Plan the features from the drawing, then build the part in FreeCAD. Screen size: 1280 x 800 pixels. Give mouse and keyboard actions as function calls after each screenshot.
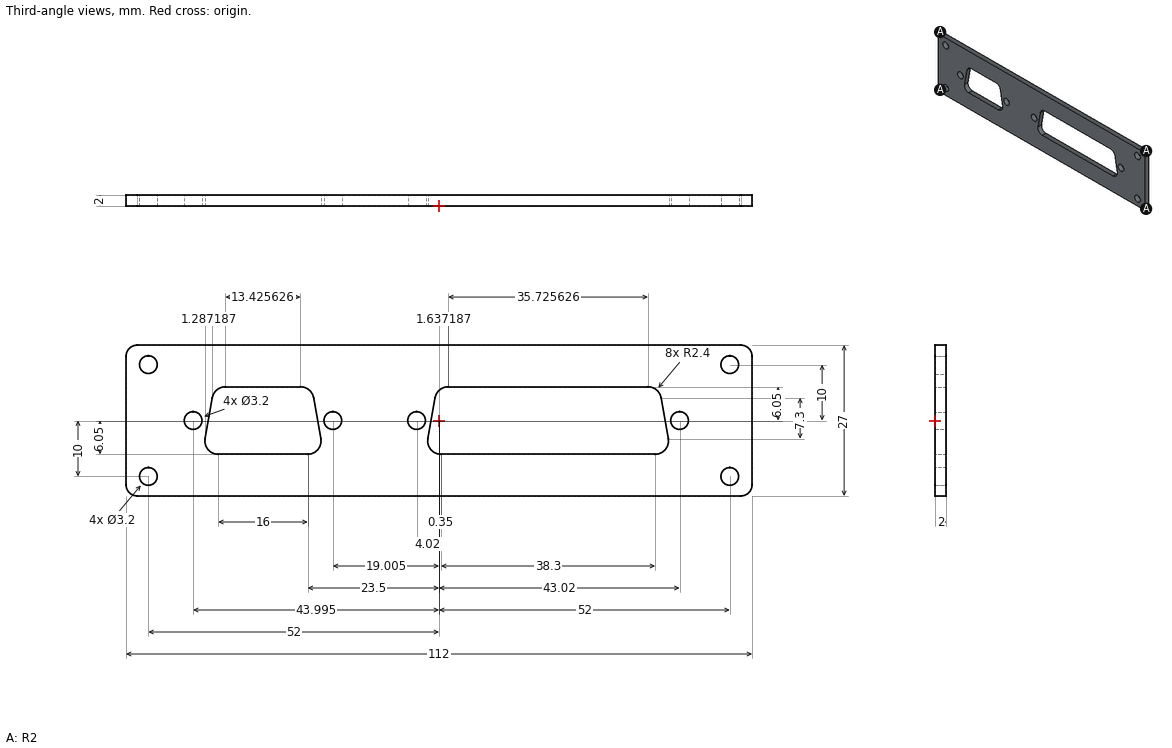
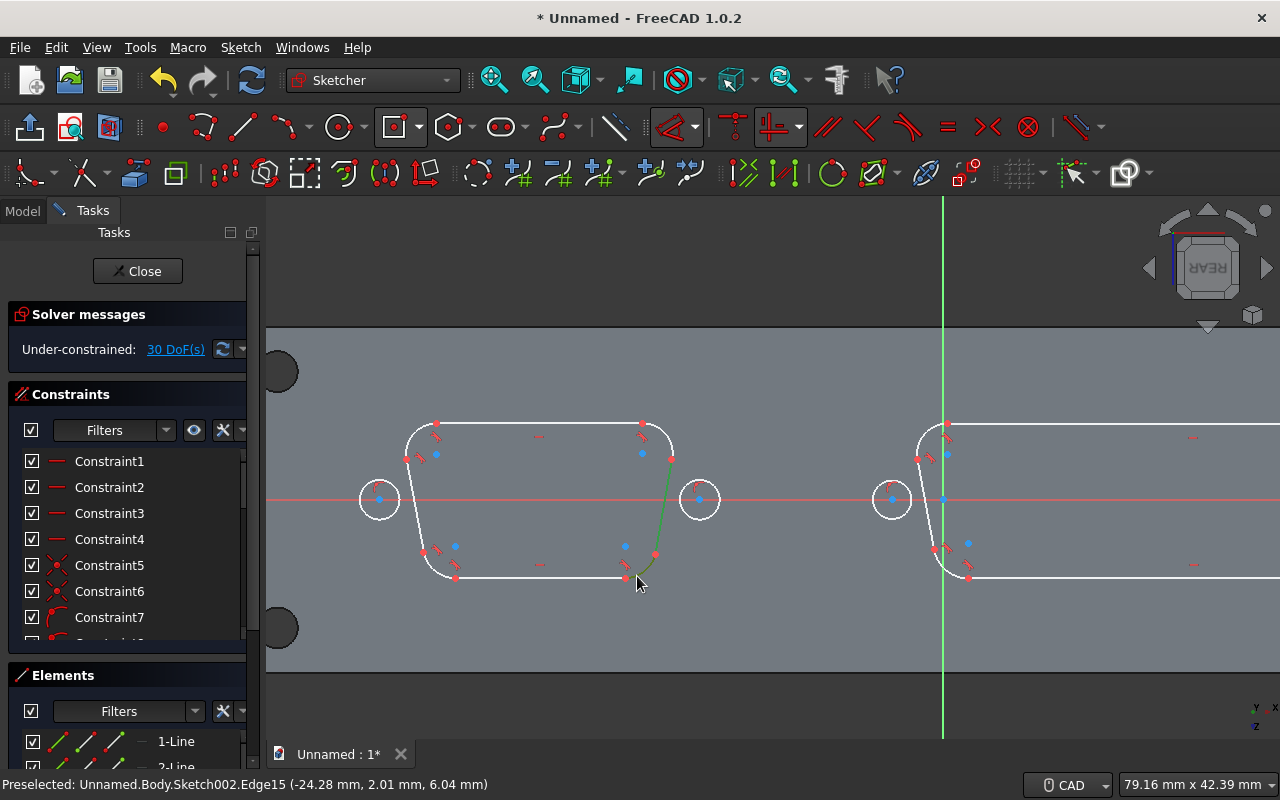
click(908, 128)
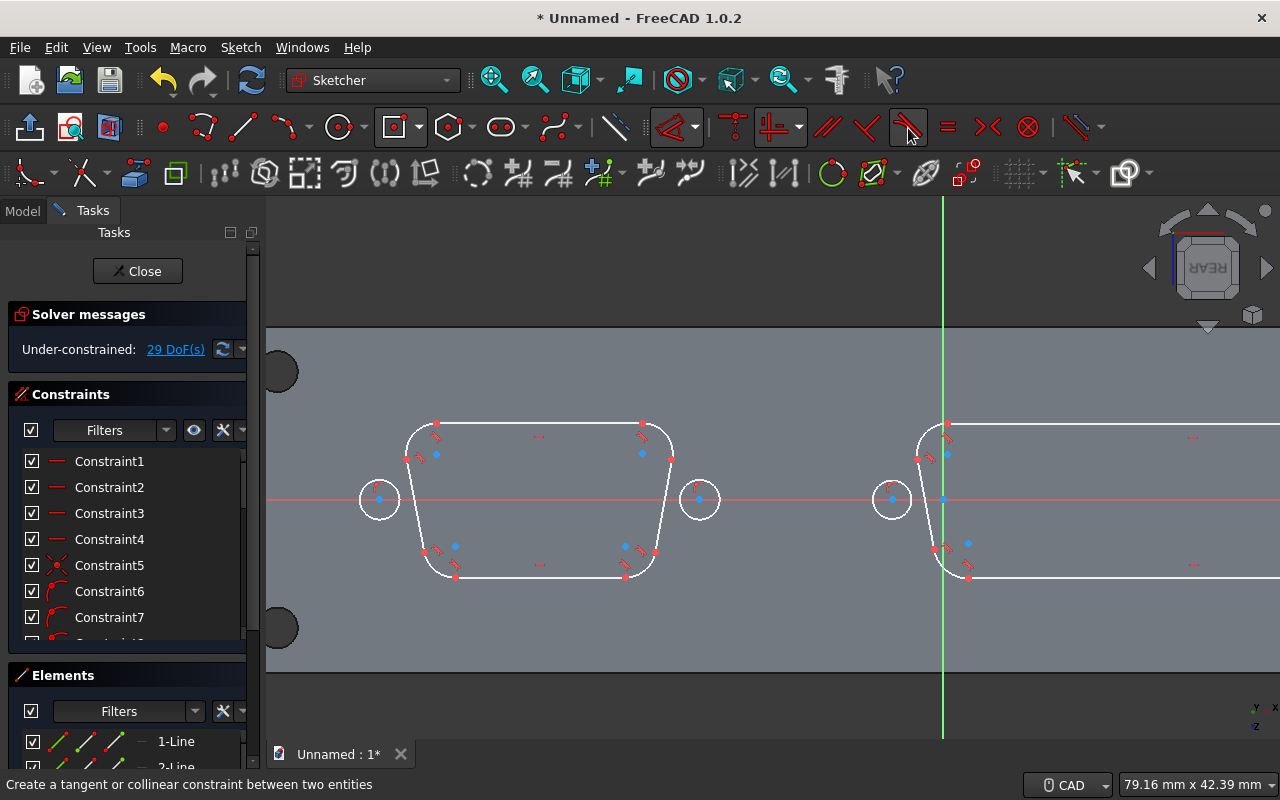
click(660, 525)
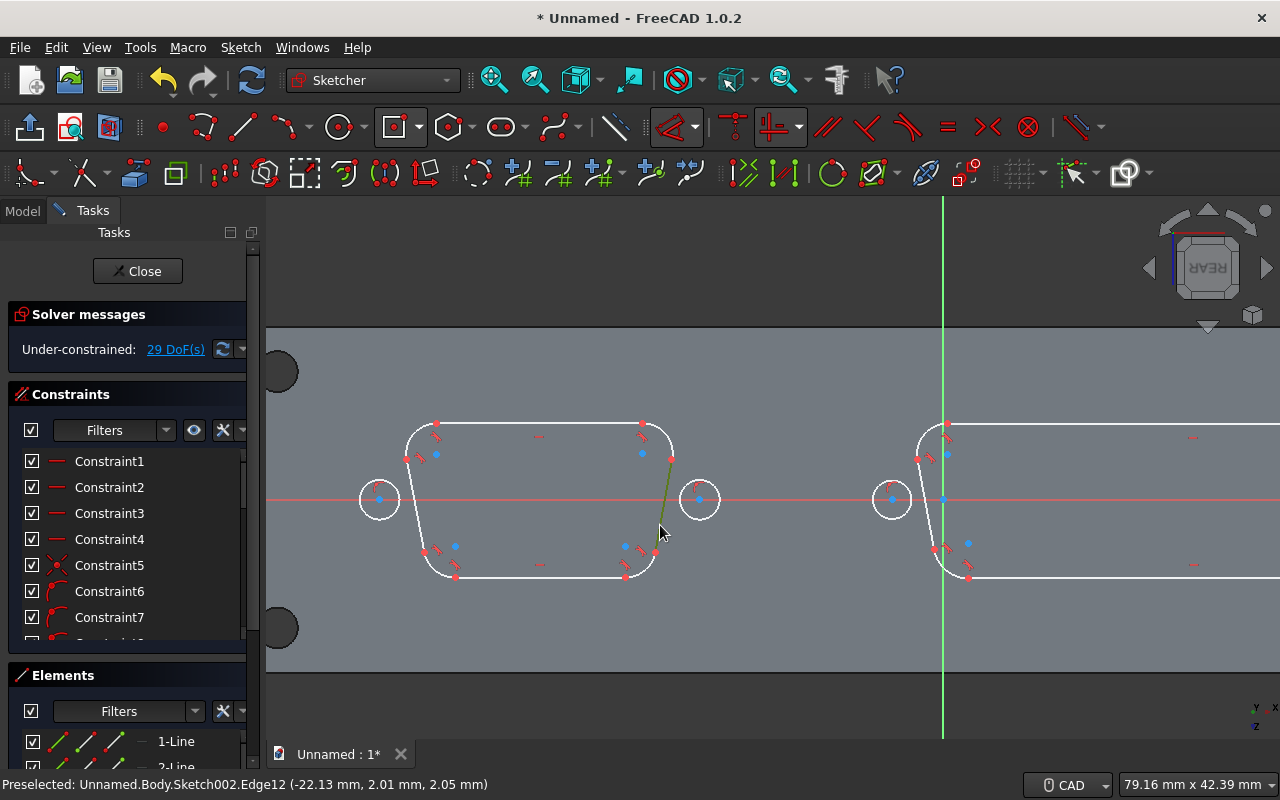
click(671, 444)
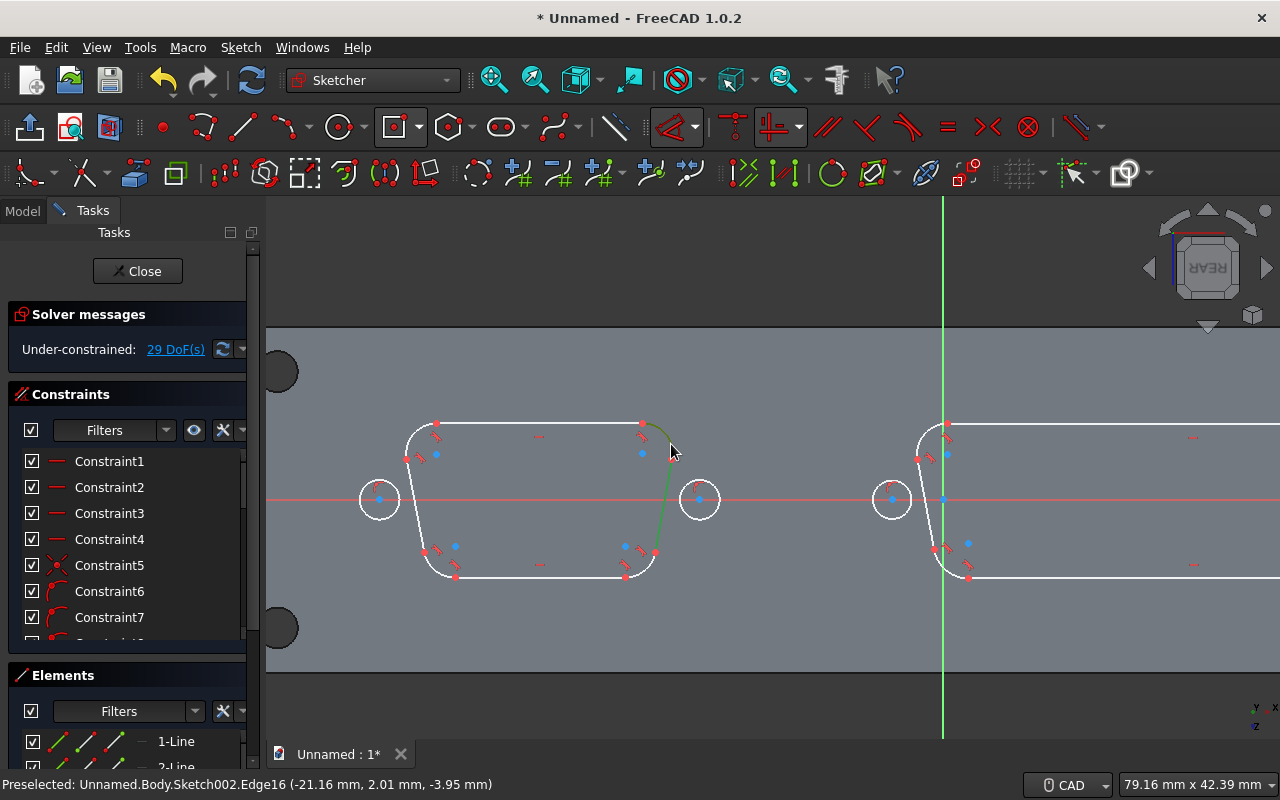
key(t)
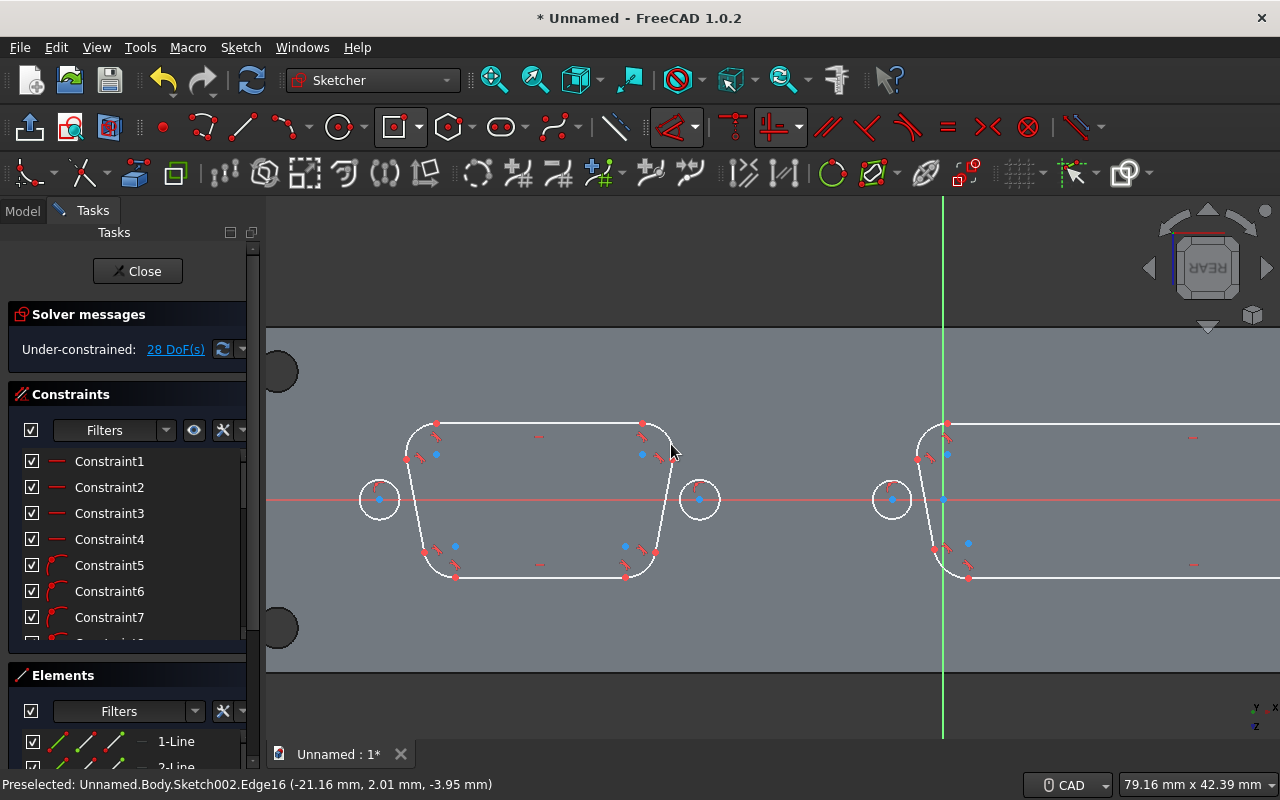
scroll(421, 428, down, 3)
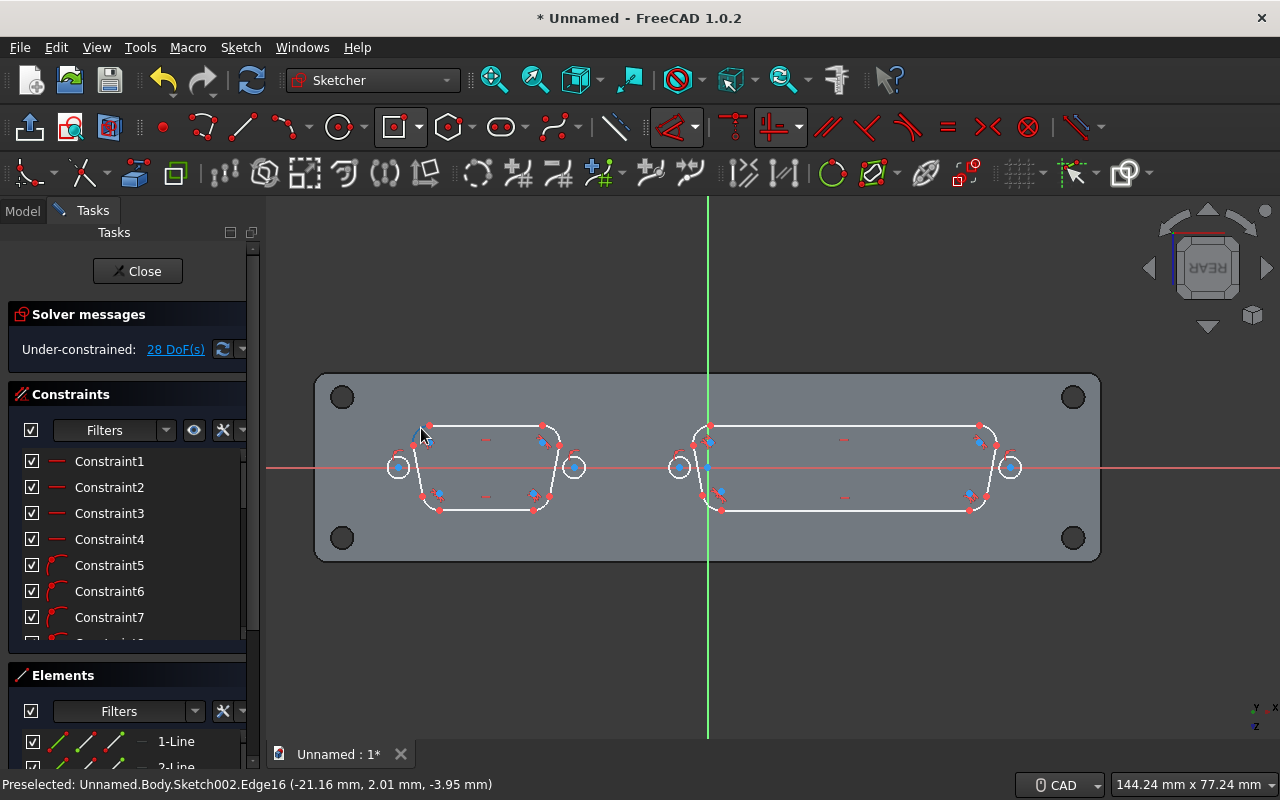
scroll(977, 509, up, 4)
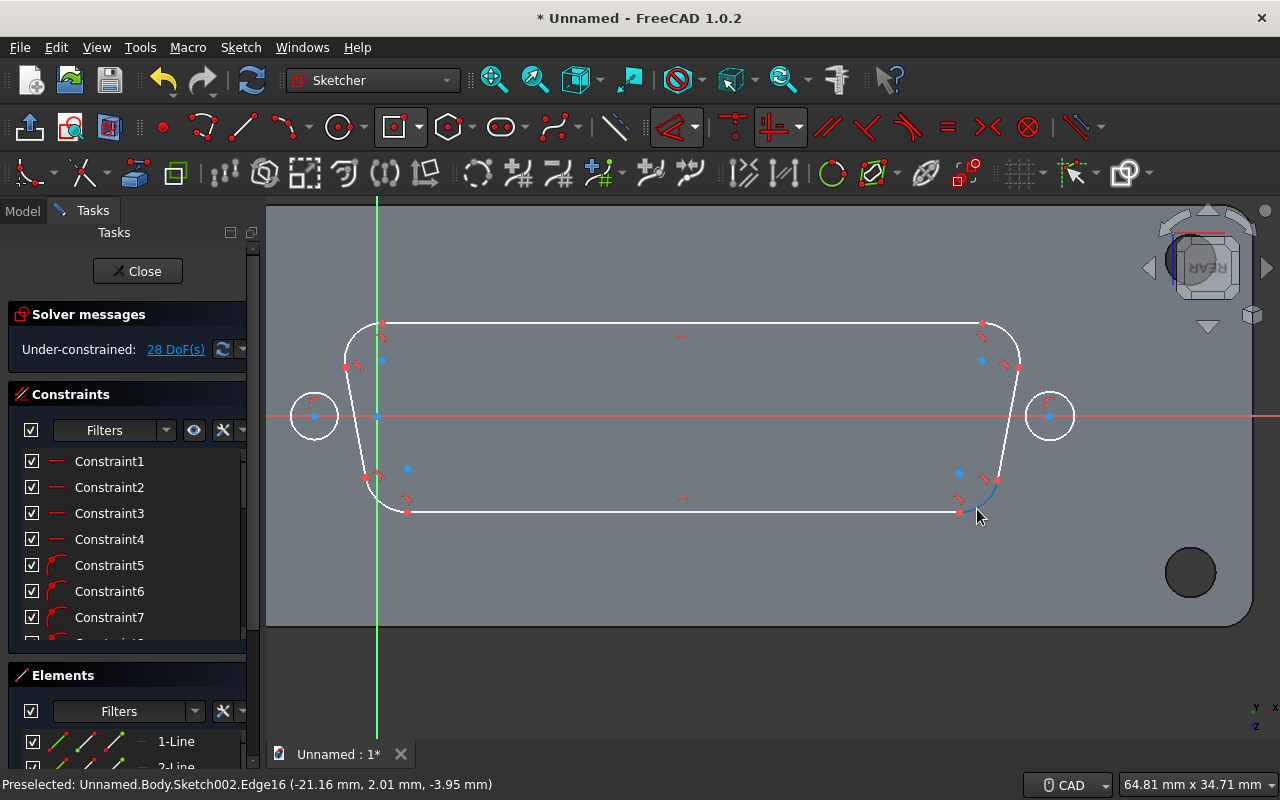
click(975, 509)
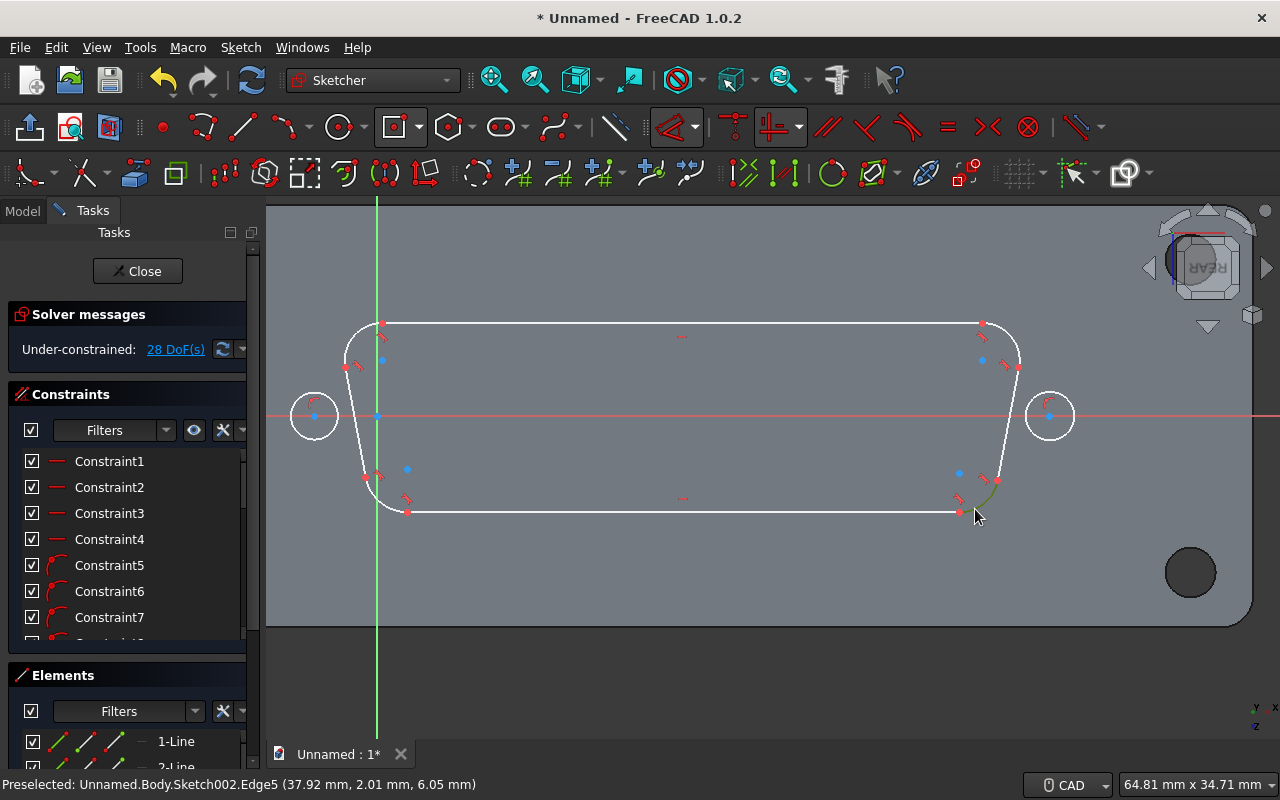
click(1017, 348)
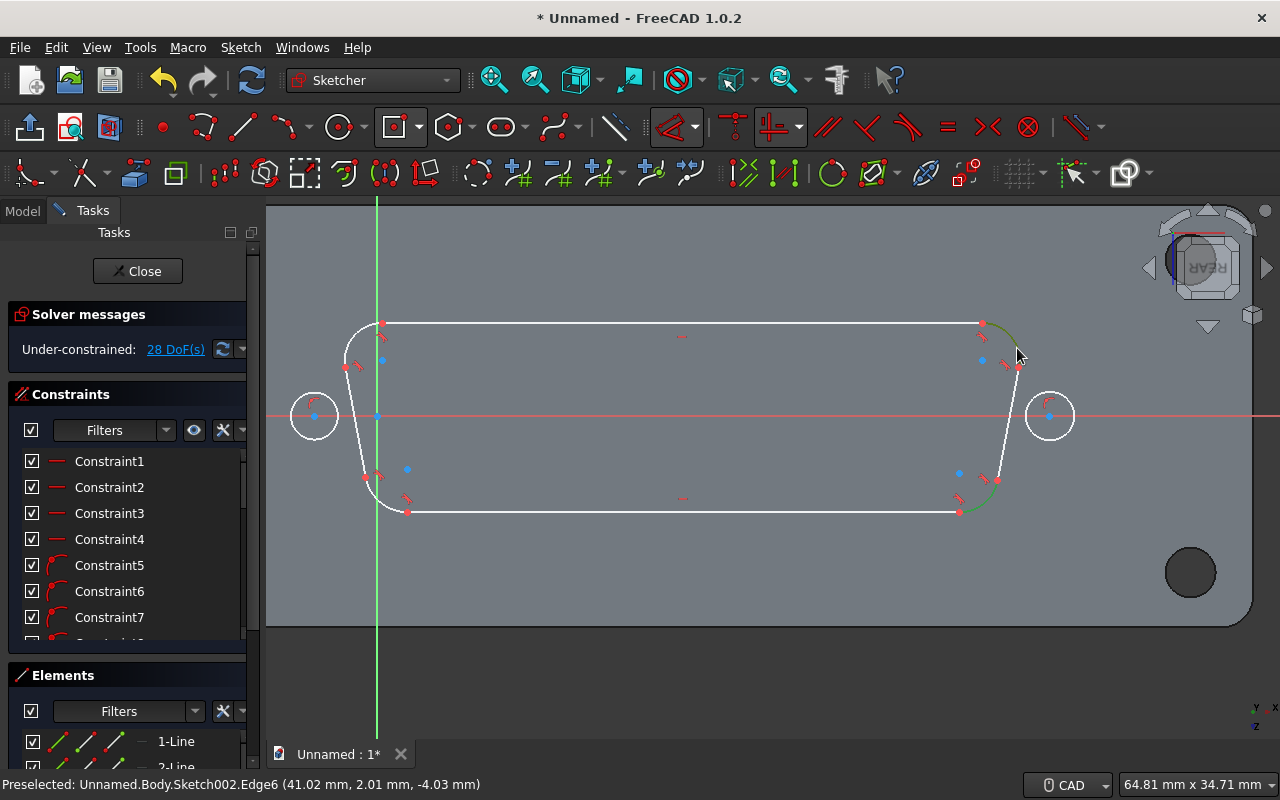
click(364, 328)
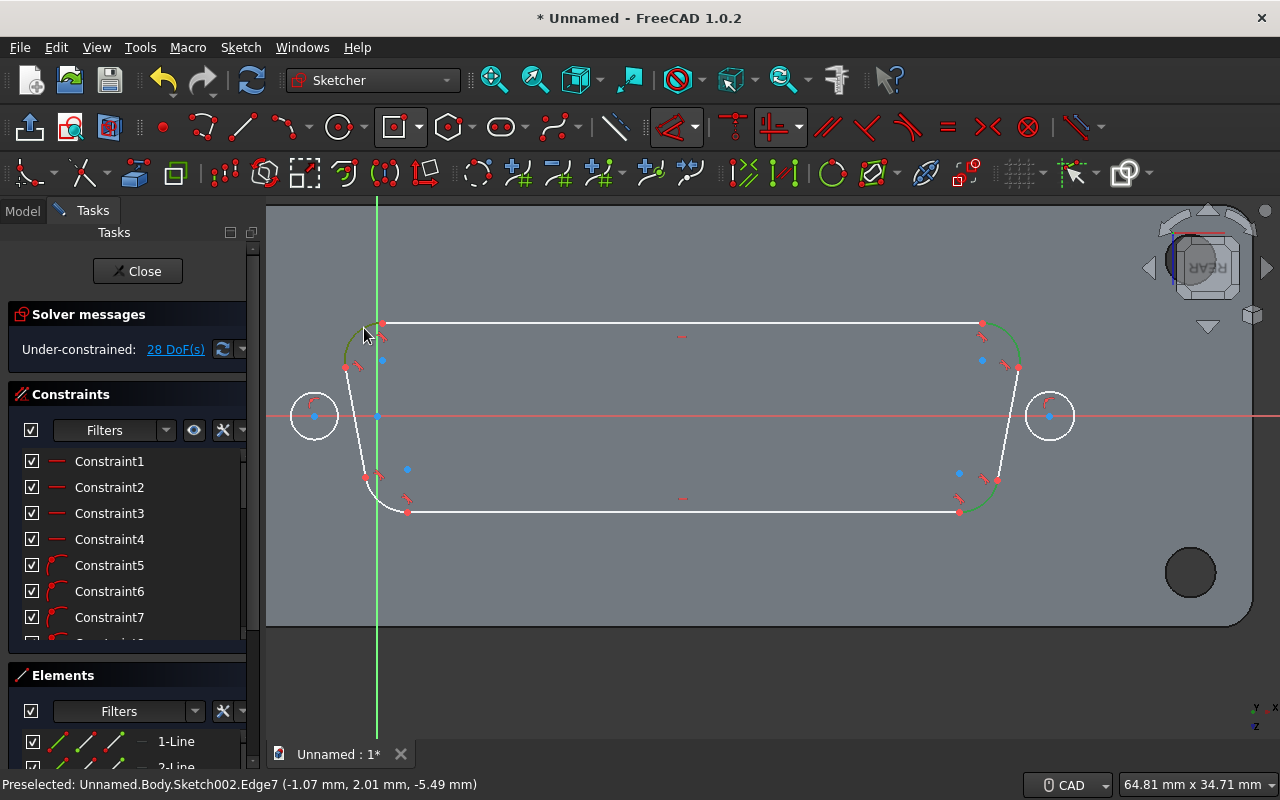
click(390, 509)